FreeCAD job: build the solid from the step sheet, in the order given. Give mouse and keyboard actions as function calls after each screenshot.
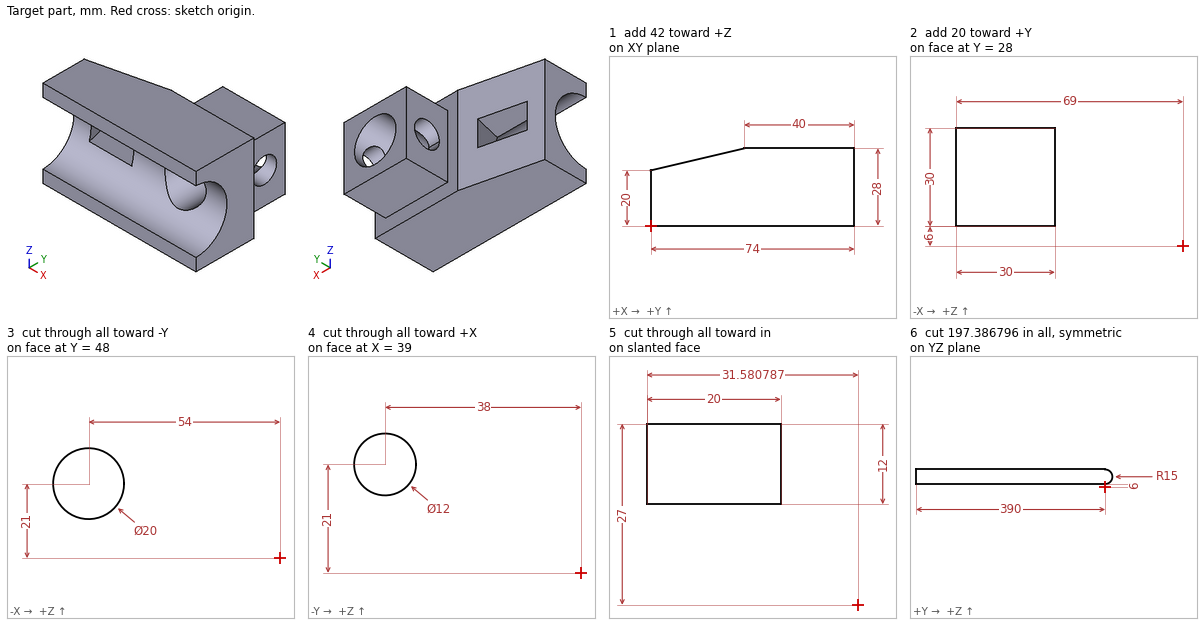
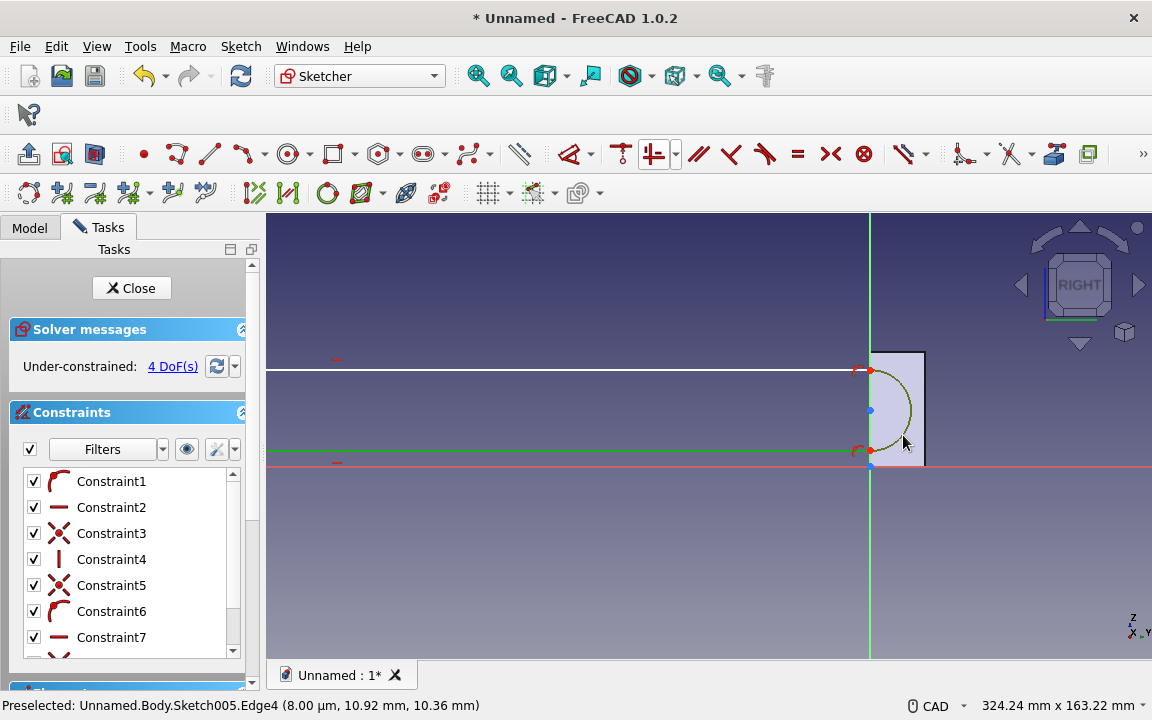
click(765, 154)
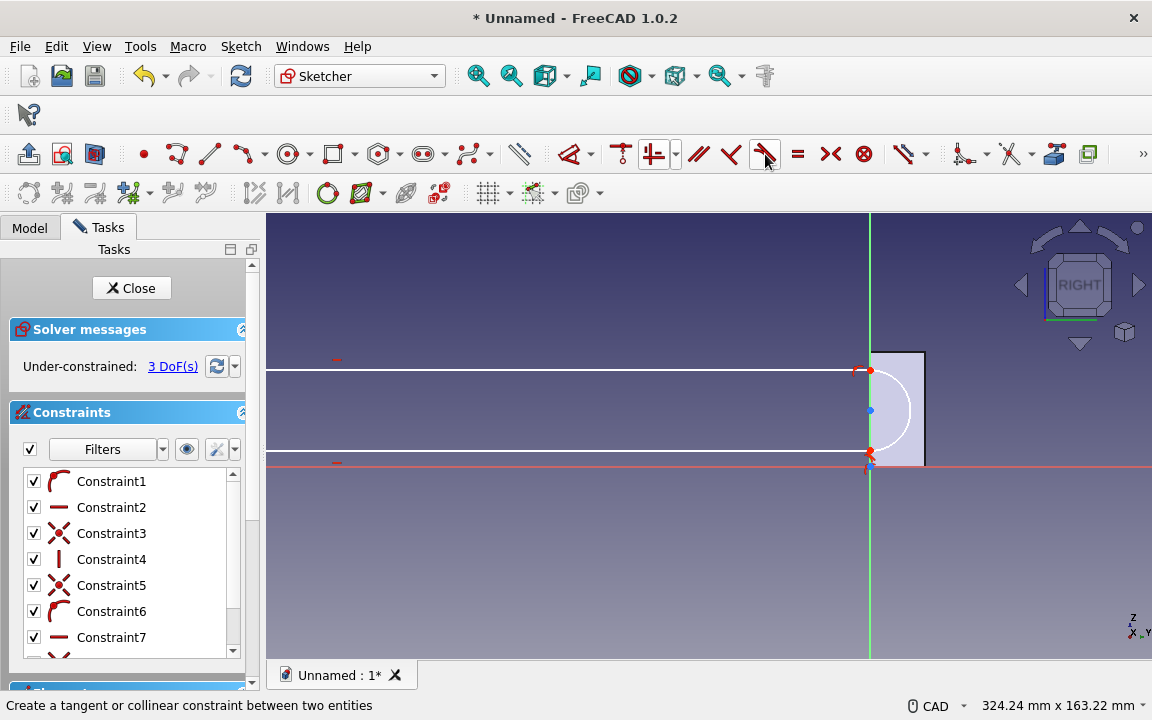
click(568, 154)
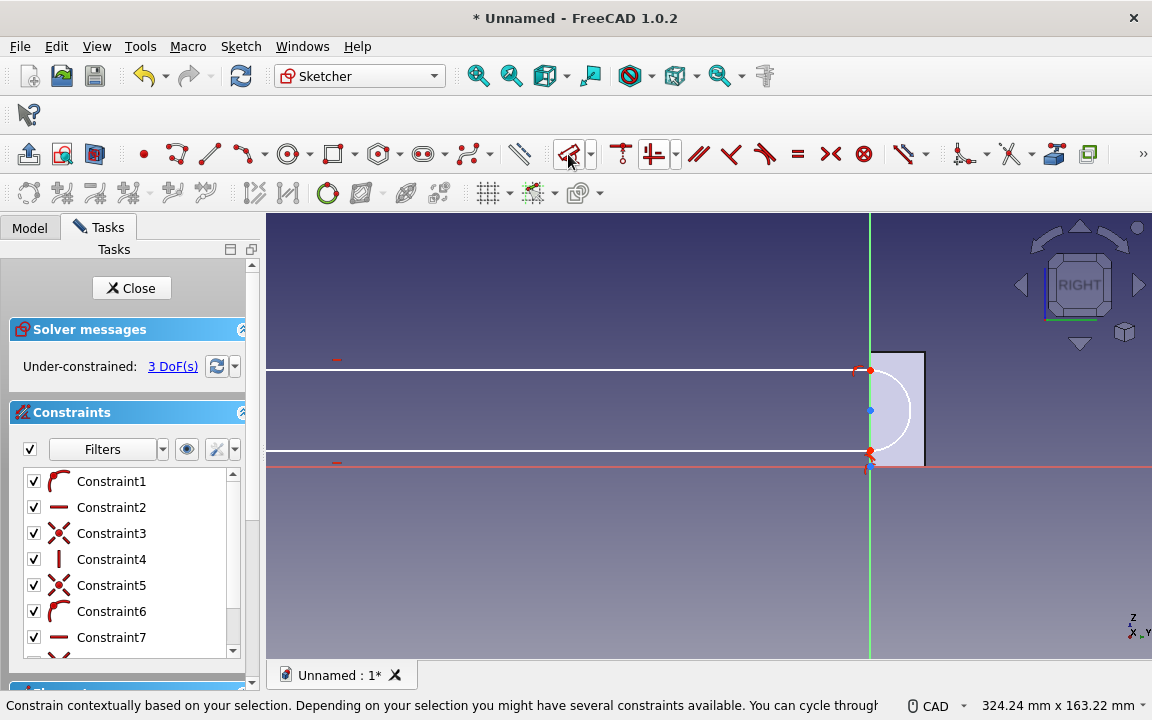
click(903, 434)
click(929, 453)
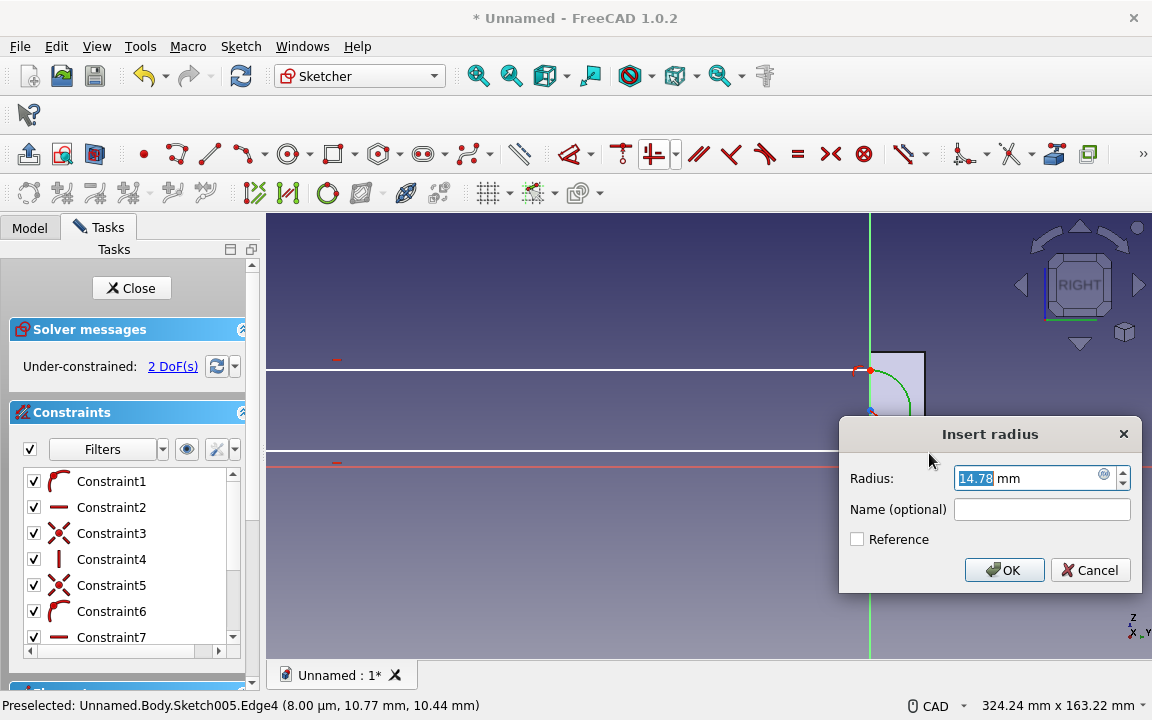
text(15)
key(Return)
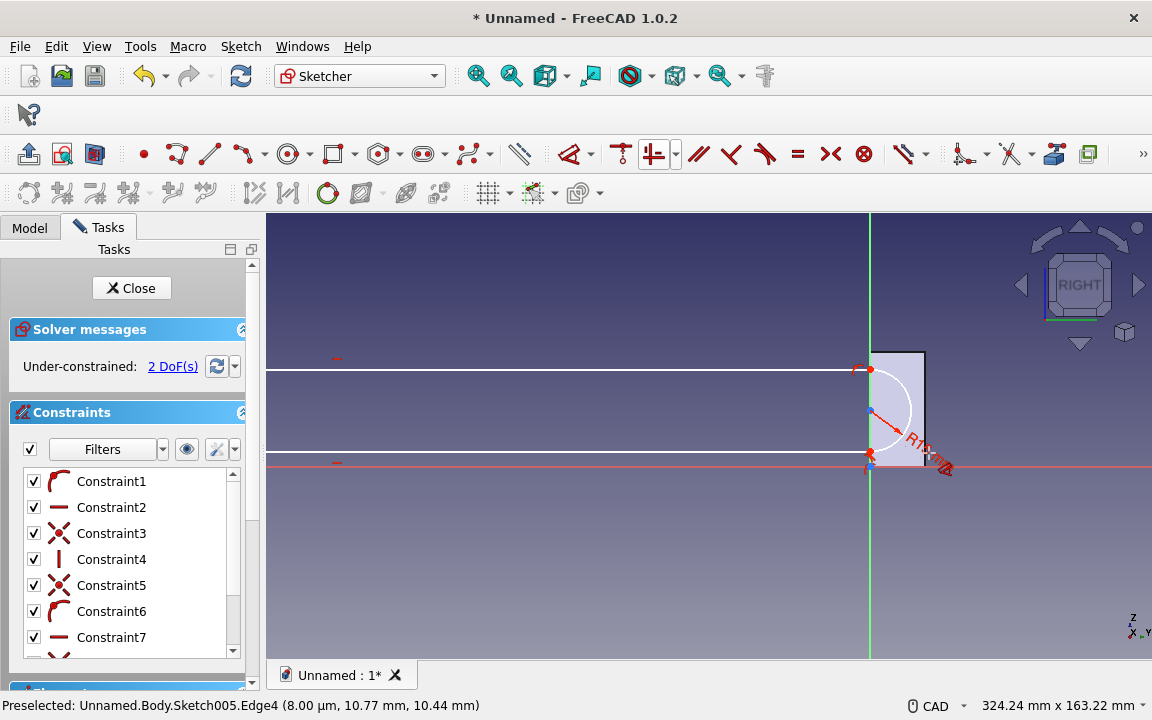
scroll(870, 452, up, 5)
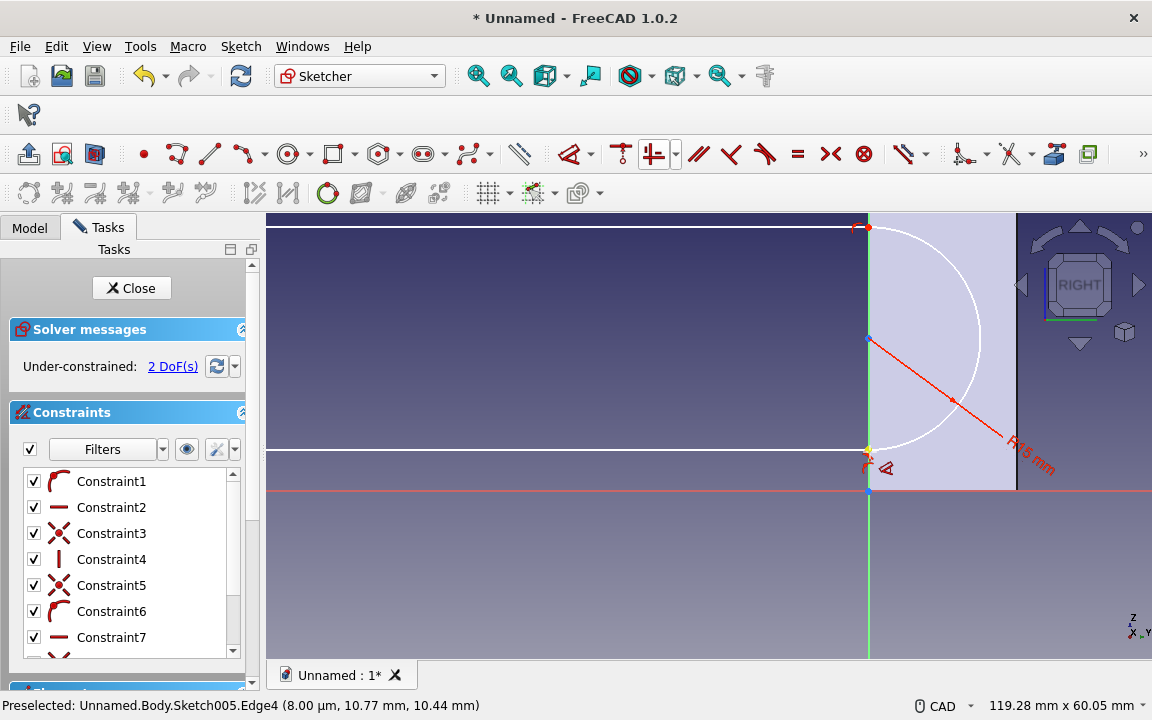
click(869, 450)
click(903, 471)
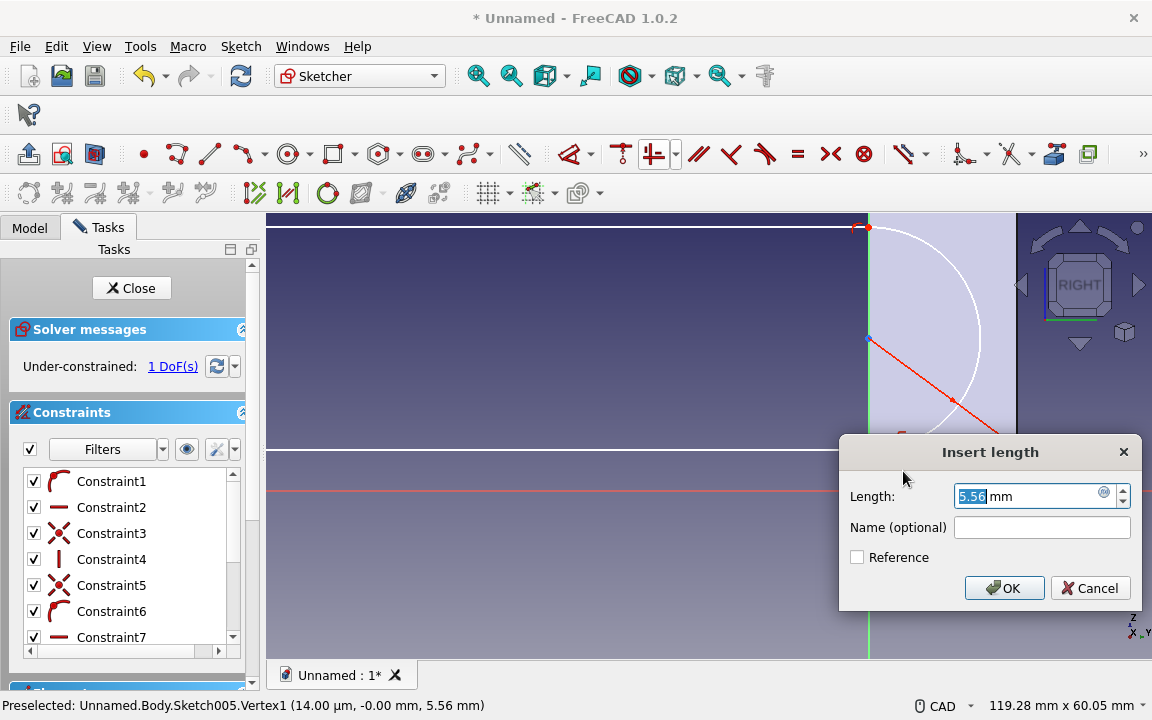
text(6)
key(Return)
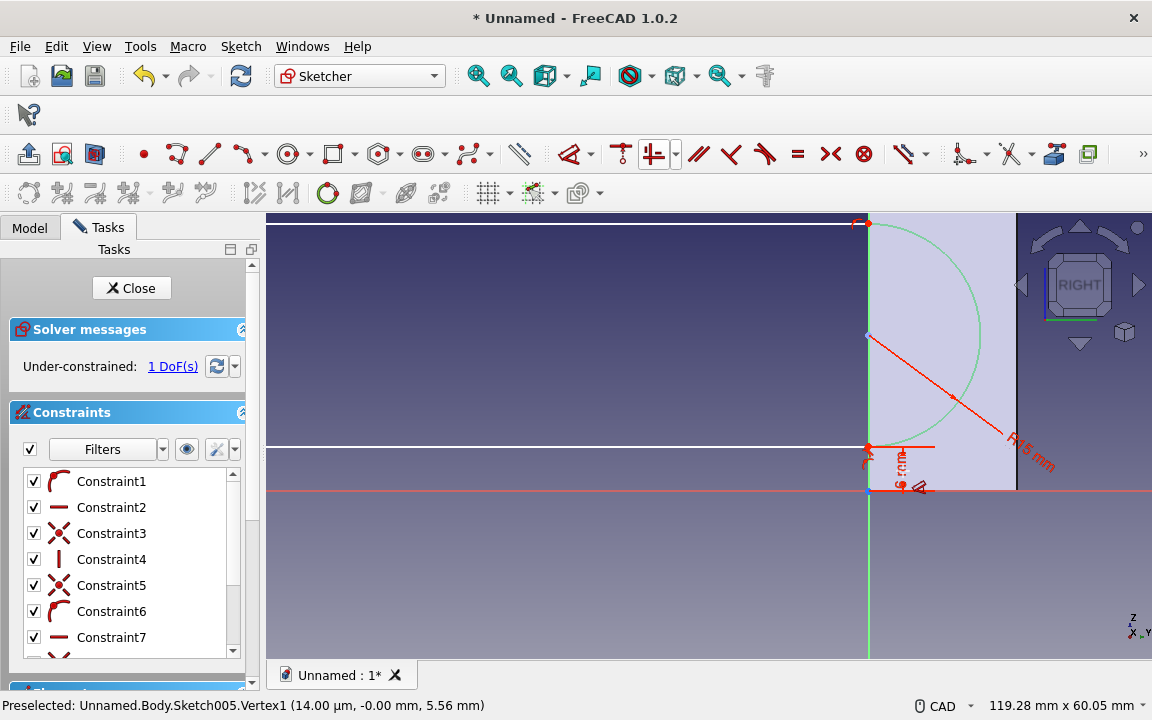
scroll(871, 452, down, 9)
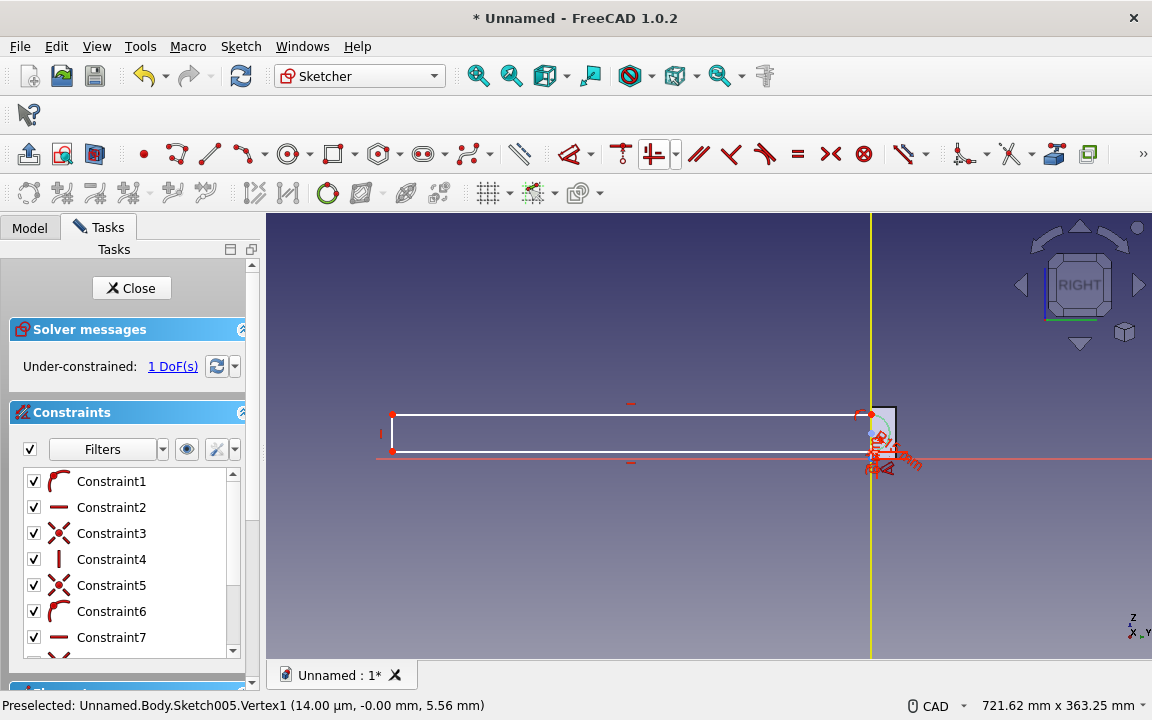
scroll(728, 452, up, 4)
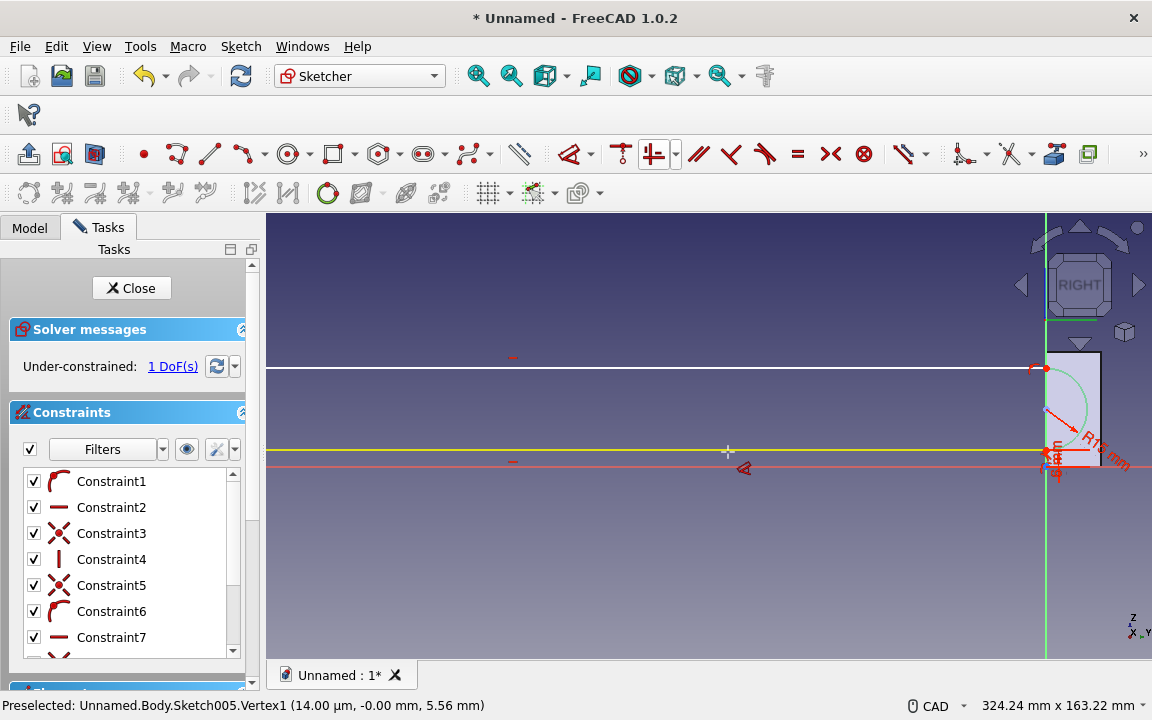
click(726, 450)
click(640, 484)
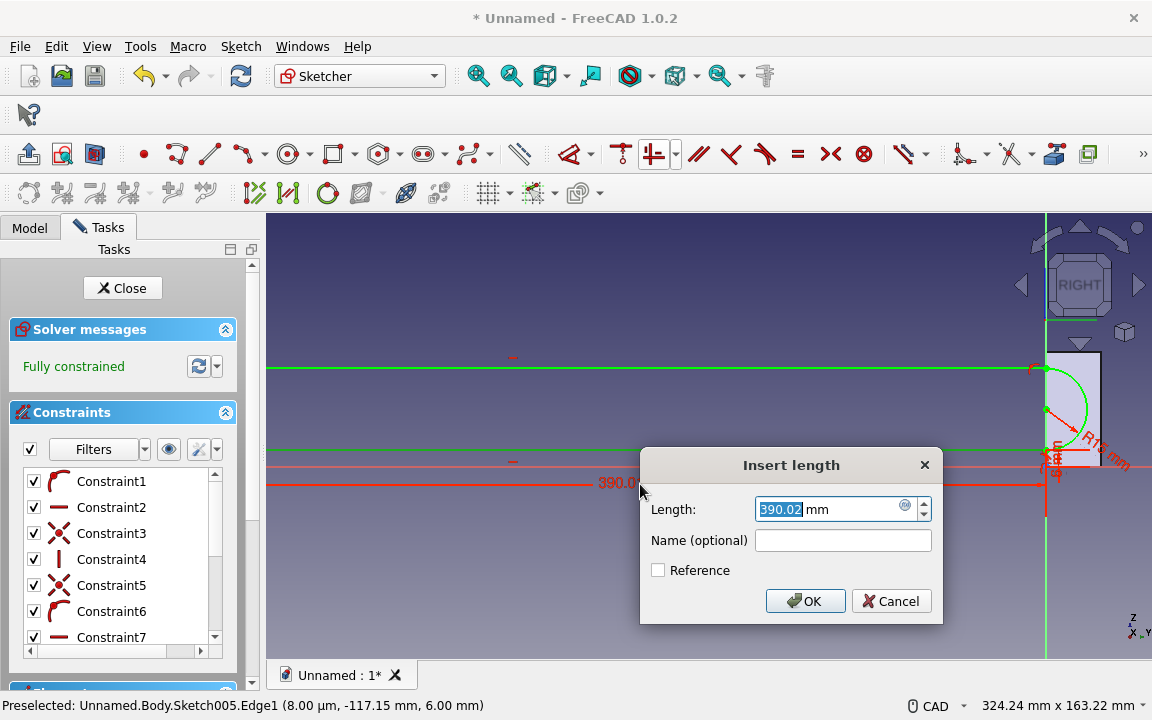
text(390)
key(Return)
key(Escape)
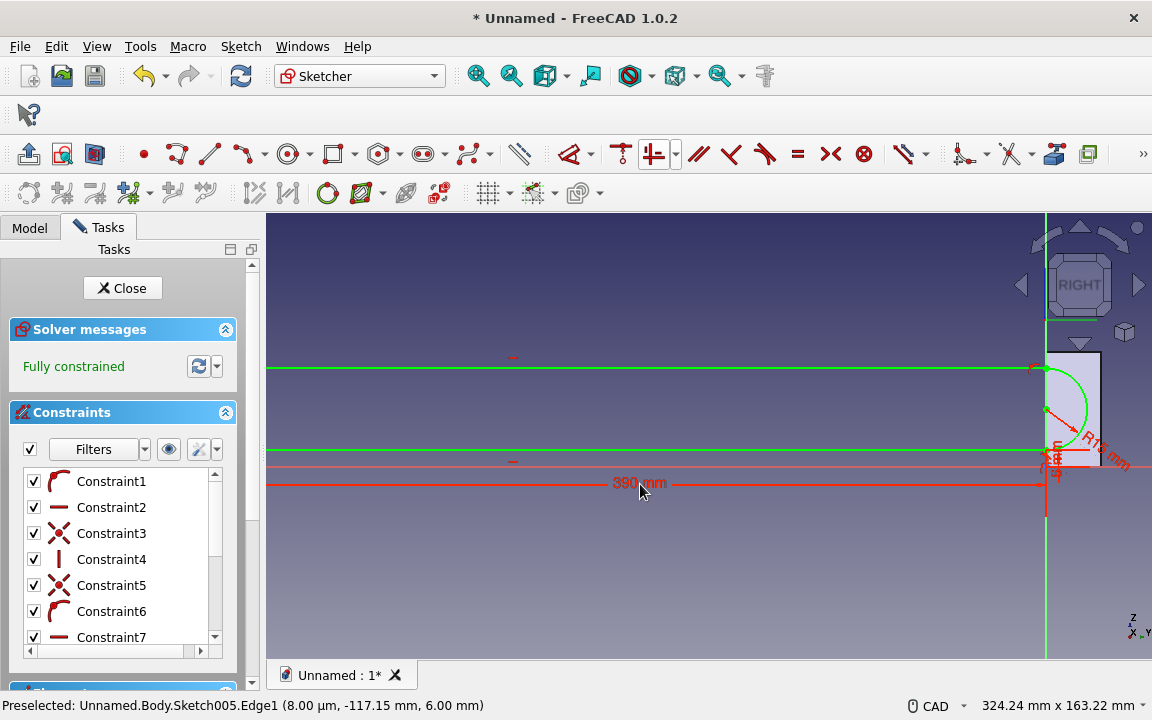
click(123, 288)